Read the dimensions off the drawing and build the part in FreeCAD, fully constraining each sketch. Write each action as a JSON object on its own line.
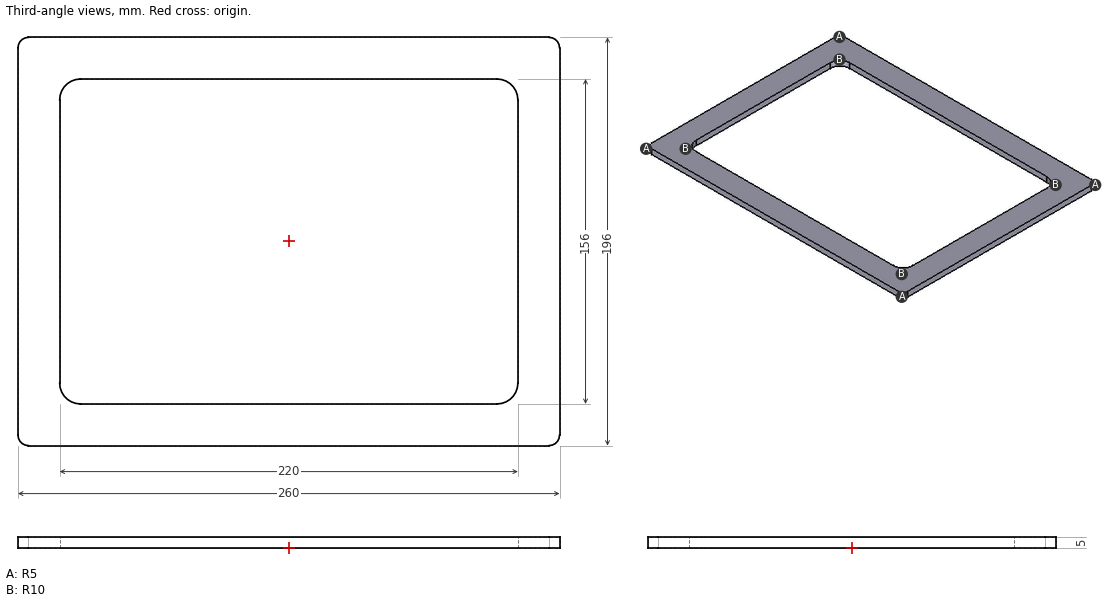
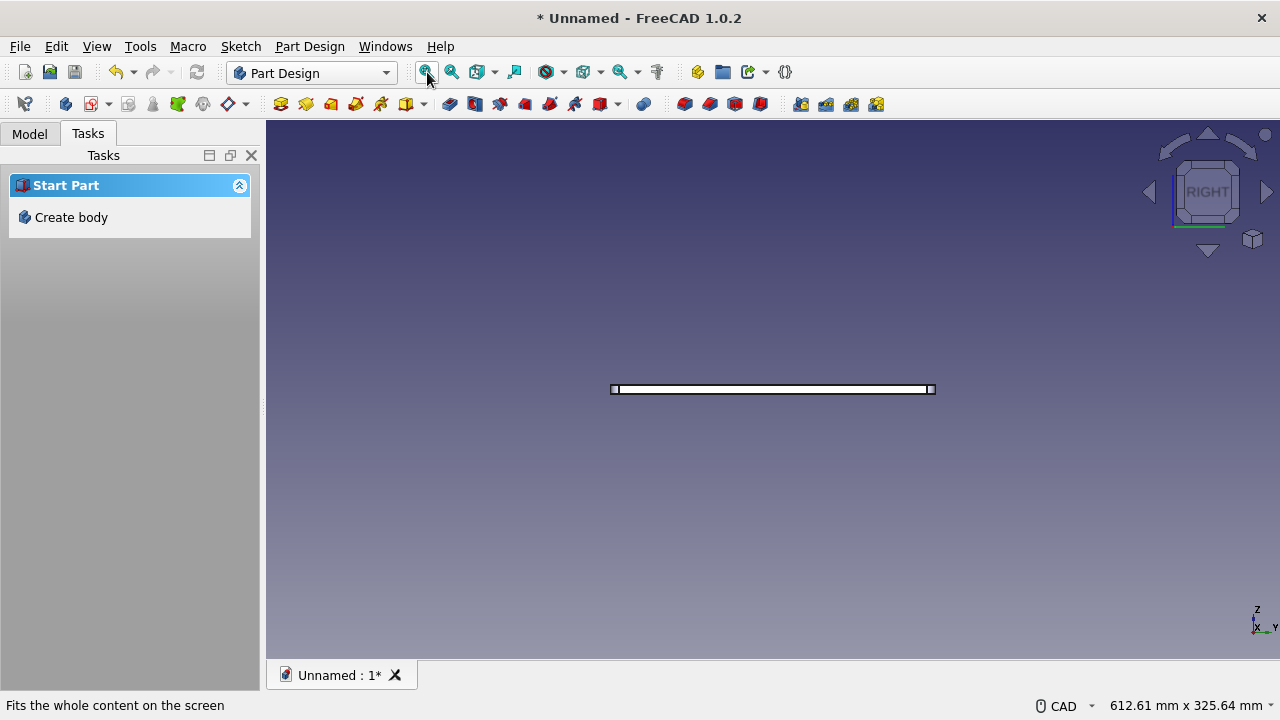
{"action": "key", "text": "5"}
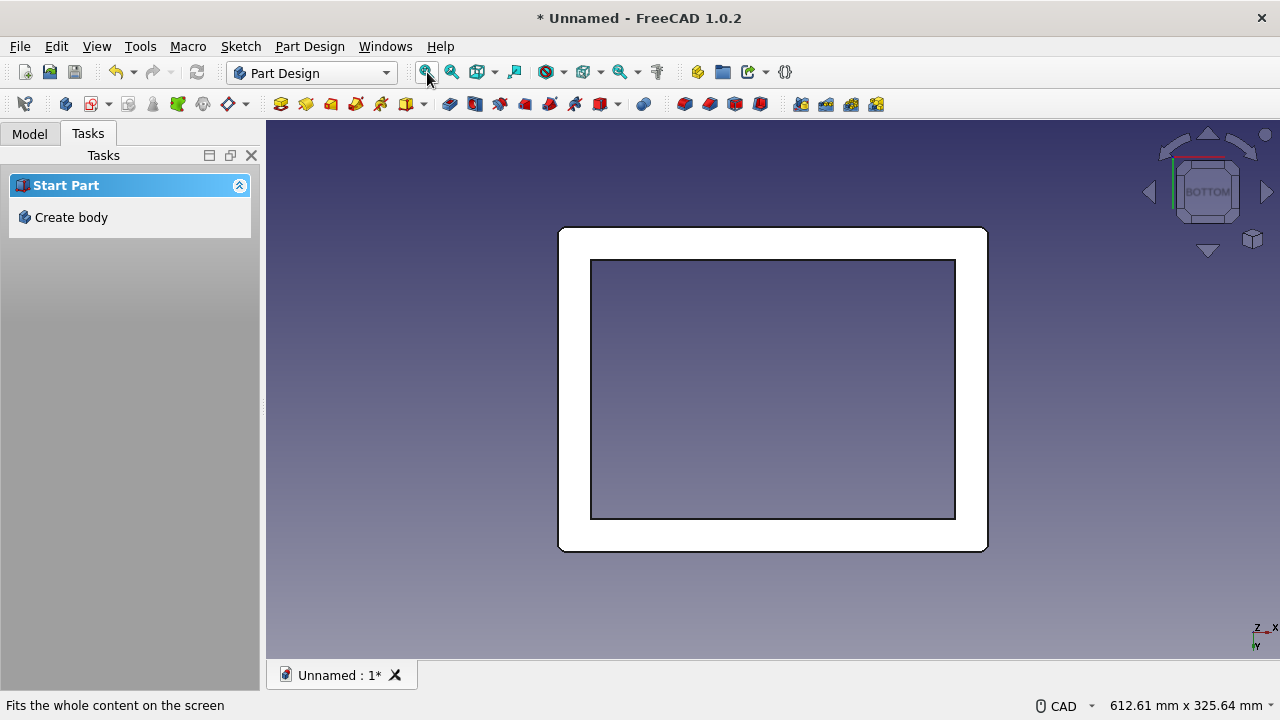
{"action": "scroll", "coordinate": [591, 518], "scroll_direction": "up", "scroll_amount": 8}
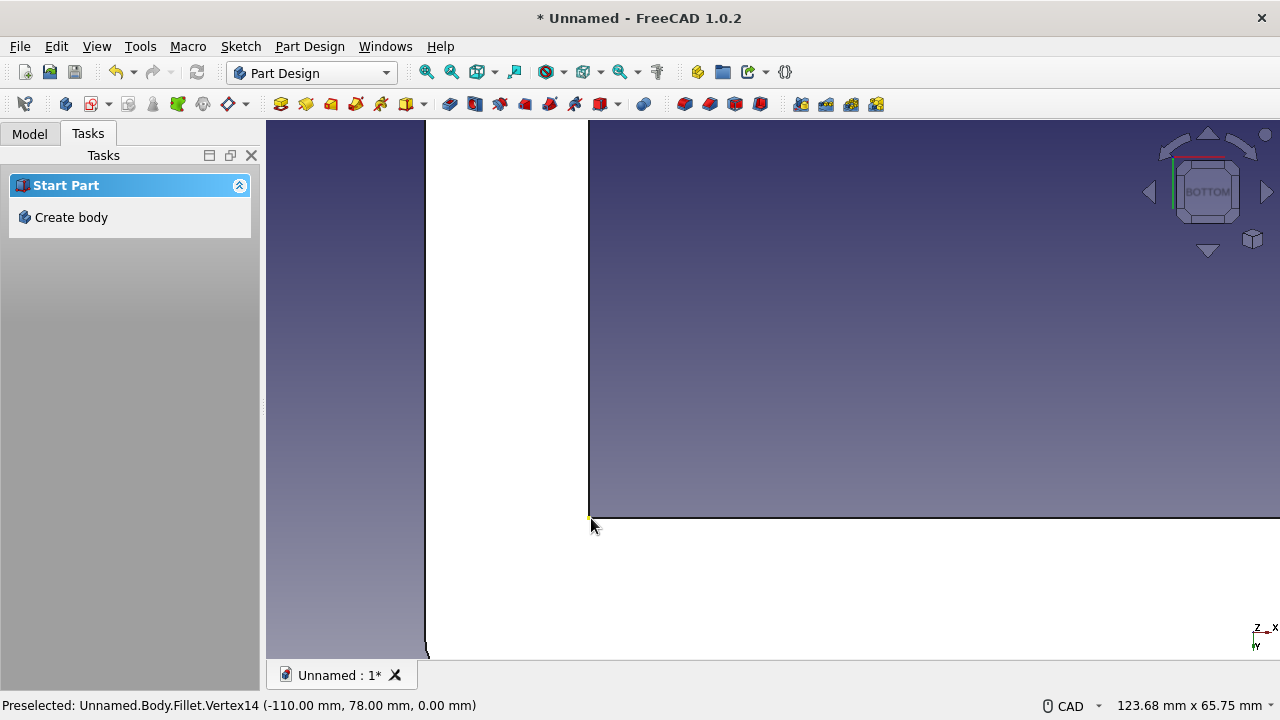
{"action": "left_click", "coordinate": [427, 72]}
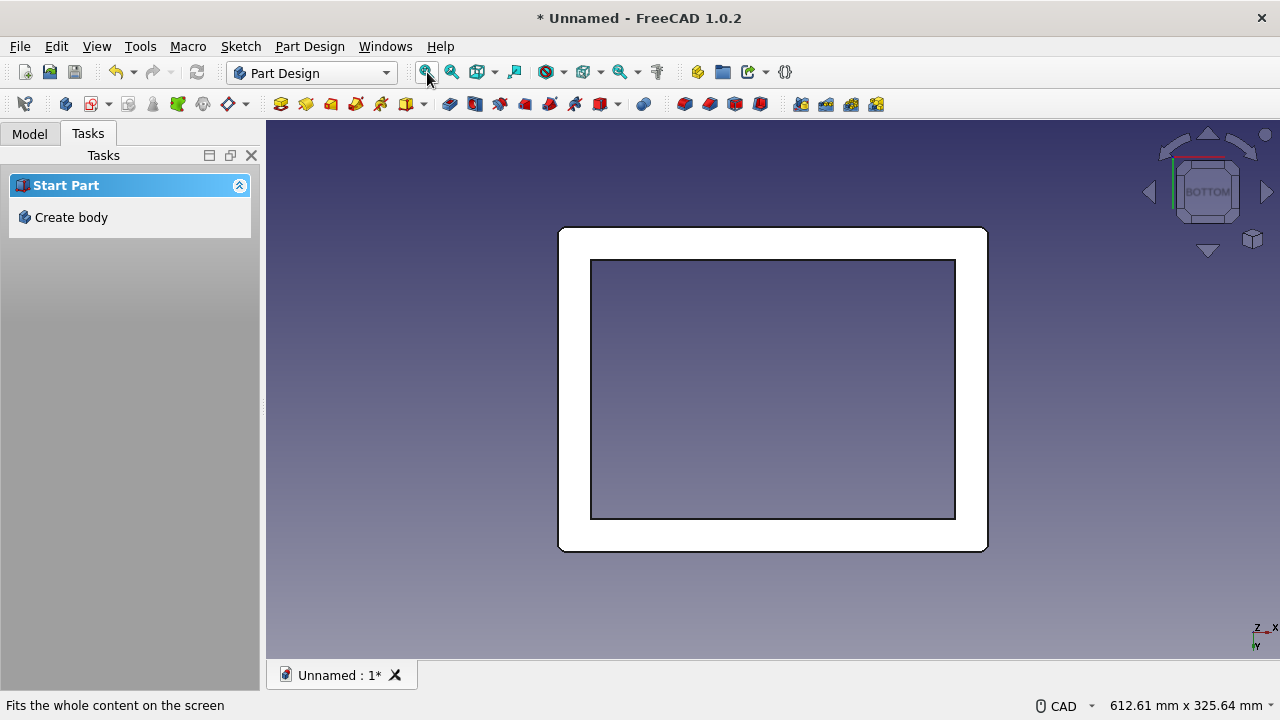
{"action": "key", "text": "4"}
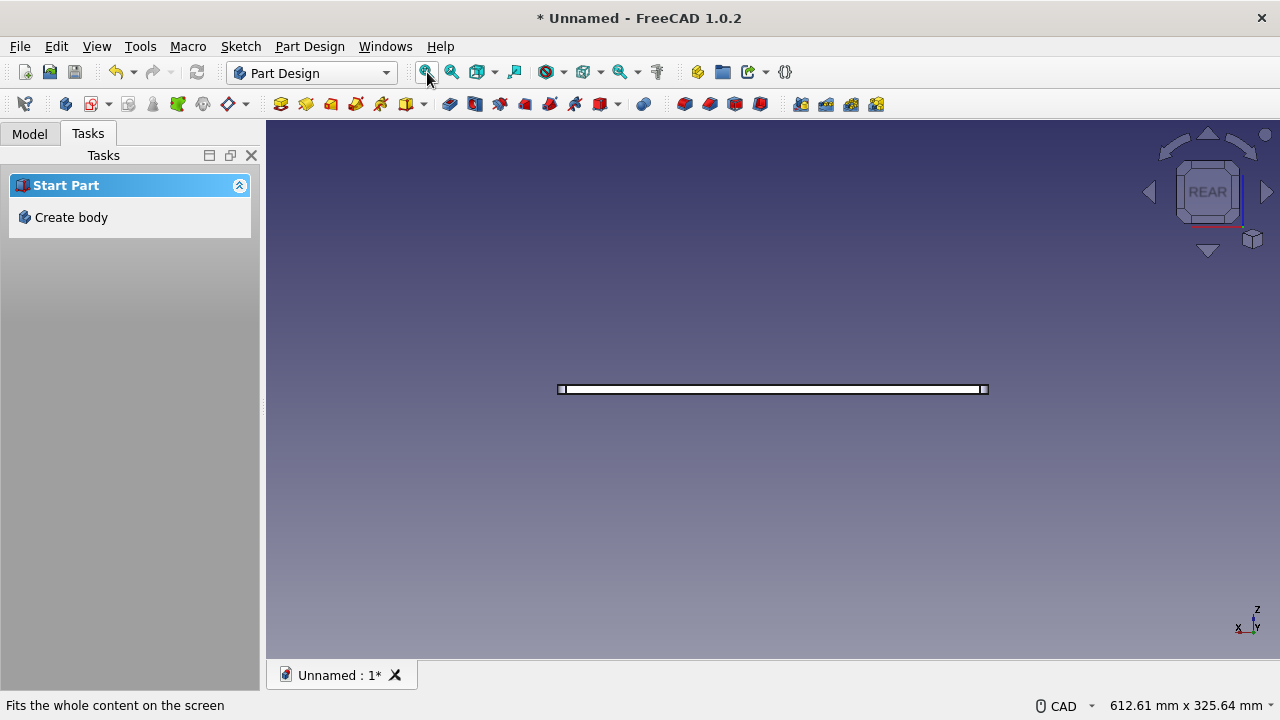
{"action": "left_click", "coordinate": [427, 72]}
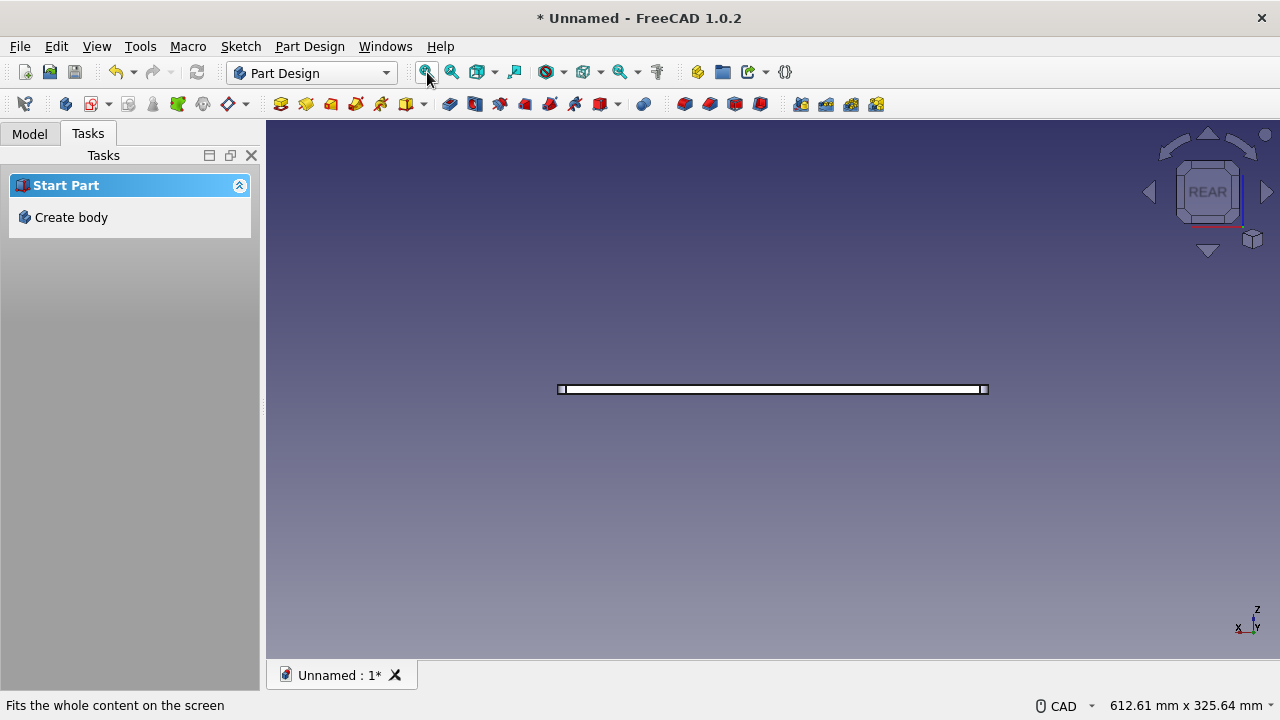
{"action": "scroll", "coordinate": [955, 389], "scroll_direction": "up", "scroll_amount": 8}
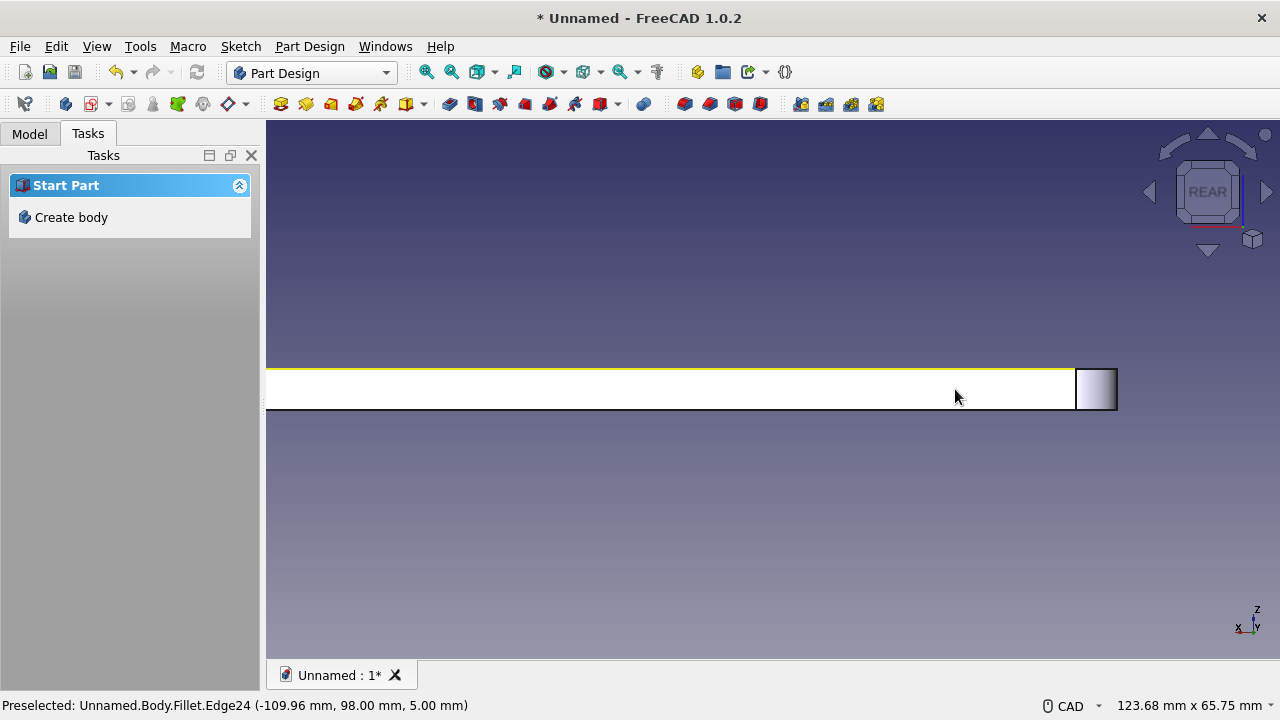
{"action": "left_click", "coordinate": [427, 72]}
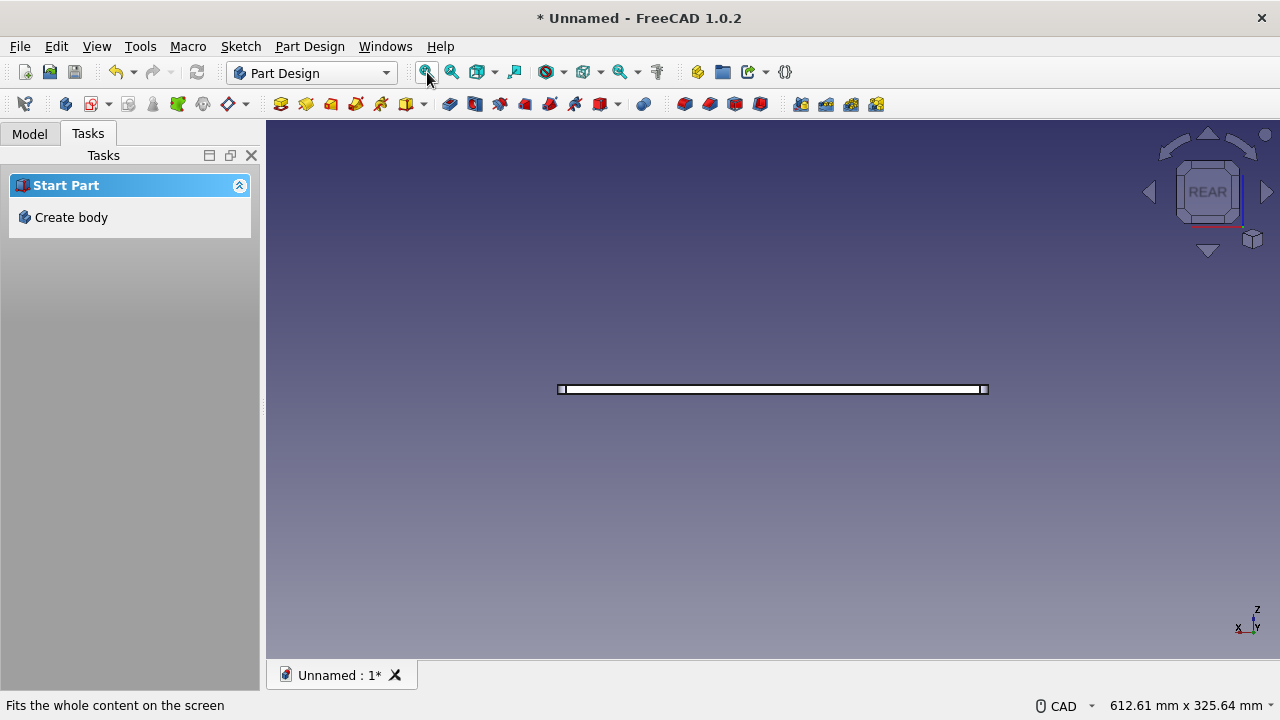
{"action": "key", "text": "6"}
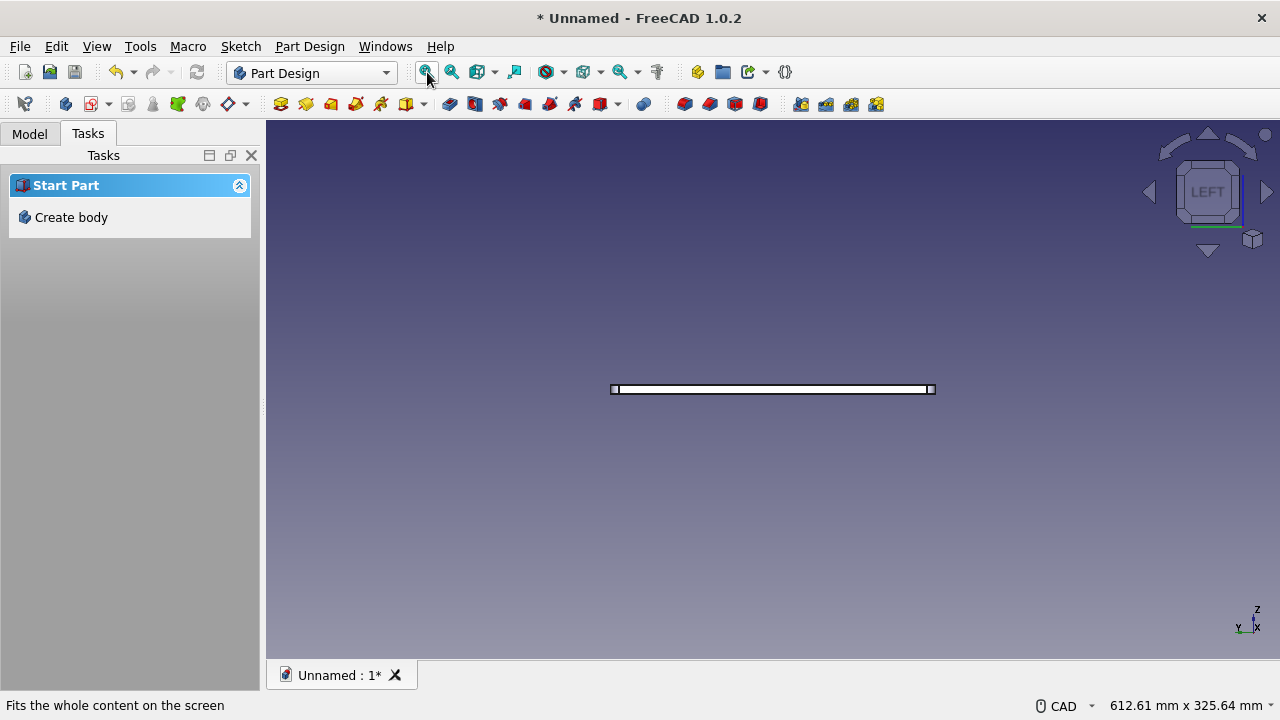
{"action": "left_click", "coordinate": [427, 72]}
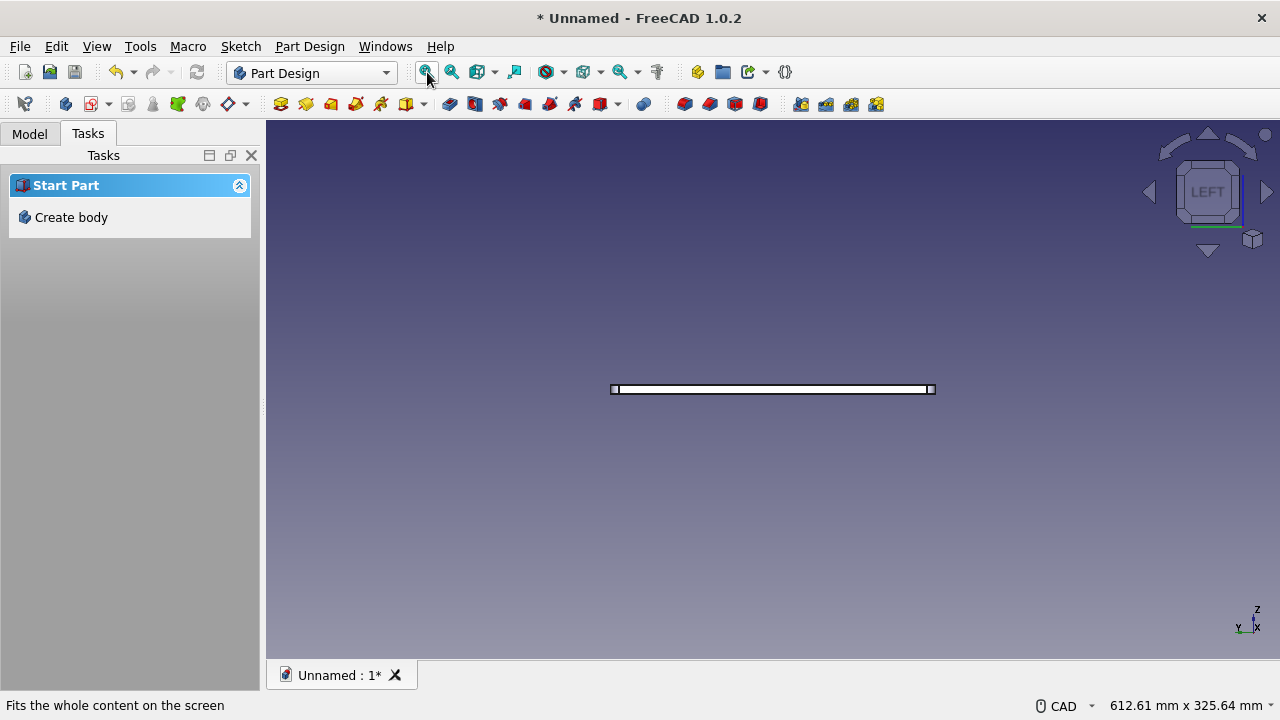
{"action": "scroll", "coordinate": [644, 388], "scroll_direction": "up", "scroll_amount": 8}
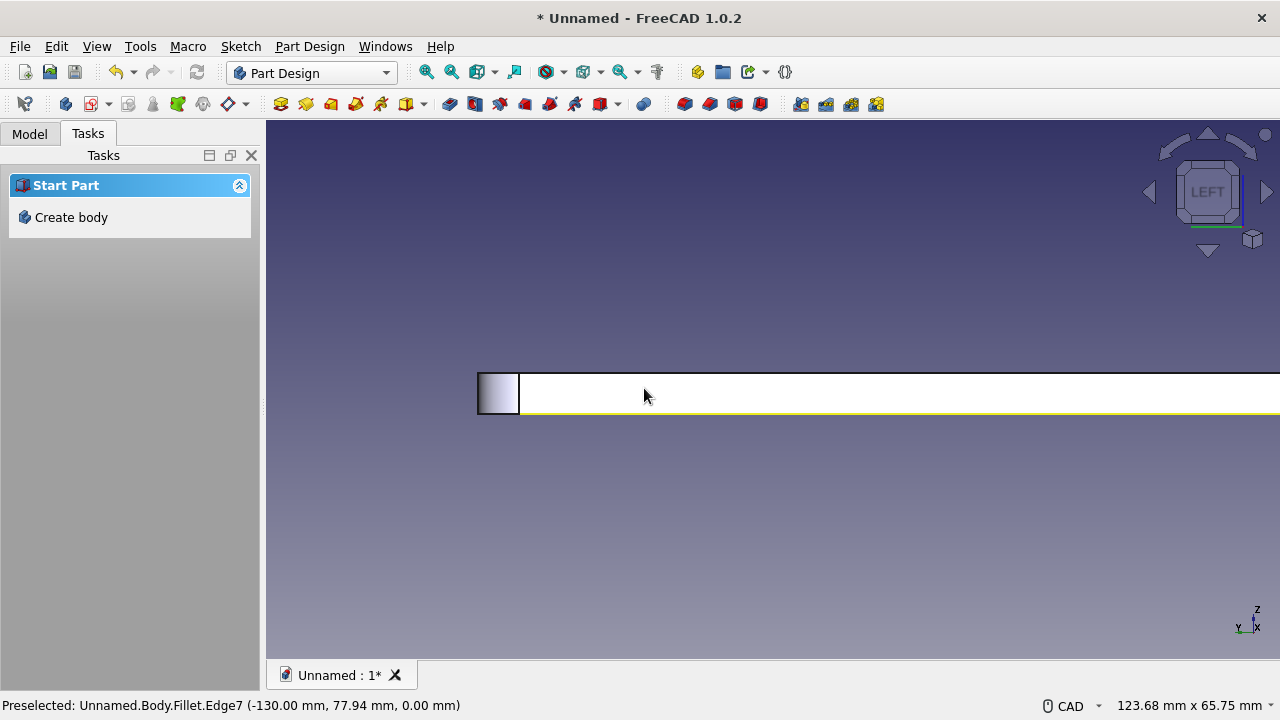
{"action": "left_click", "coordinate": [427, 72]}